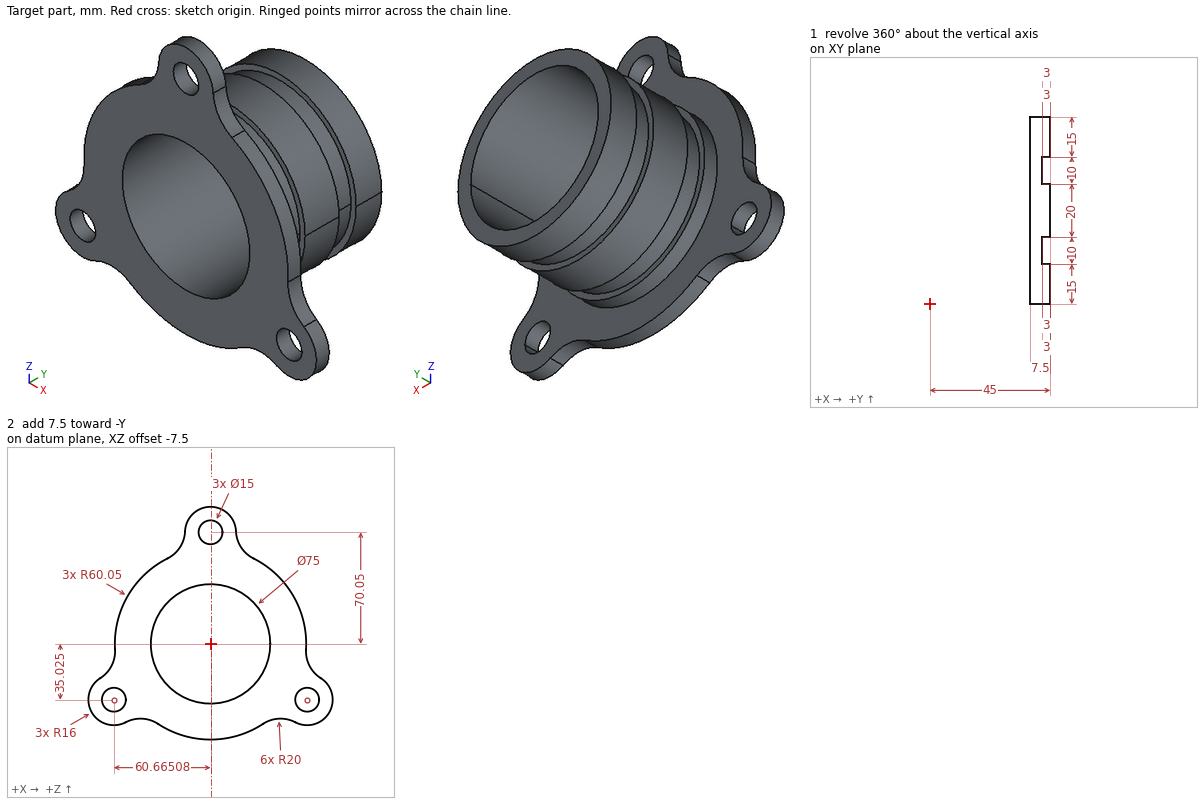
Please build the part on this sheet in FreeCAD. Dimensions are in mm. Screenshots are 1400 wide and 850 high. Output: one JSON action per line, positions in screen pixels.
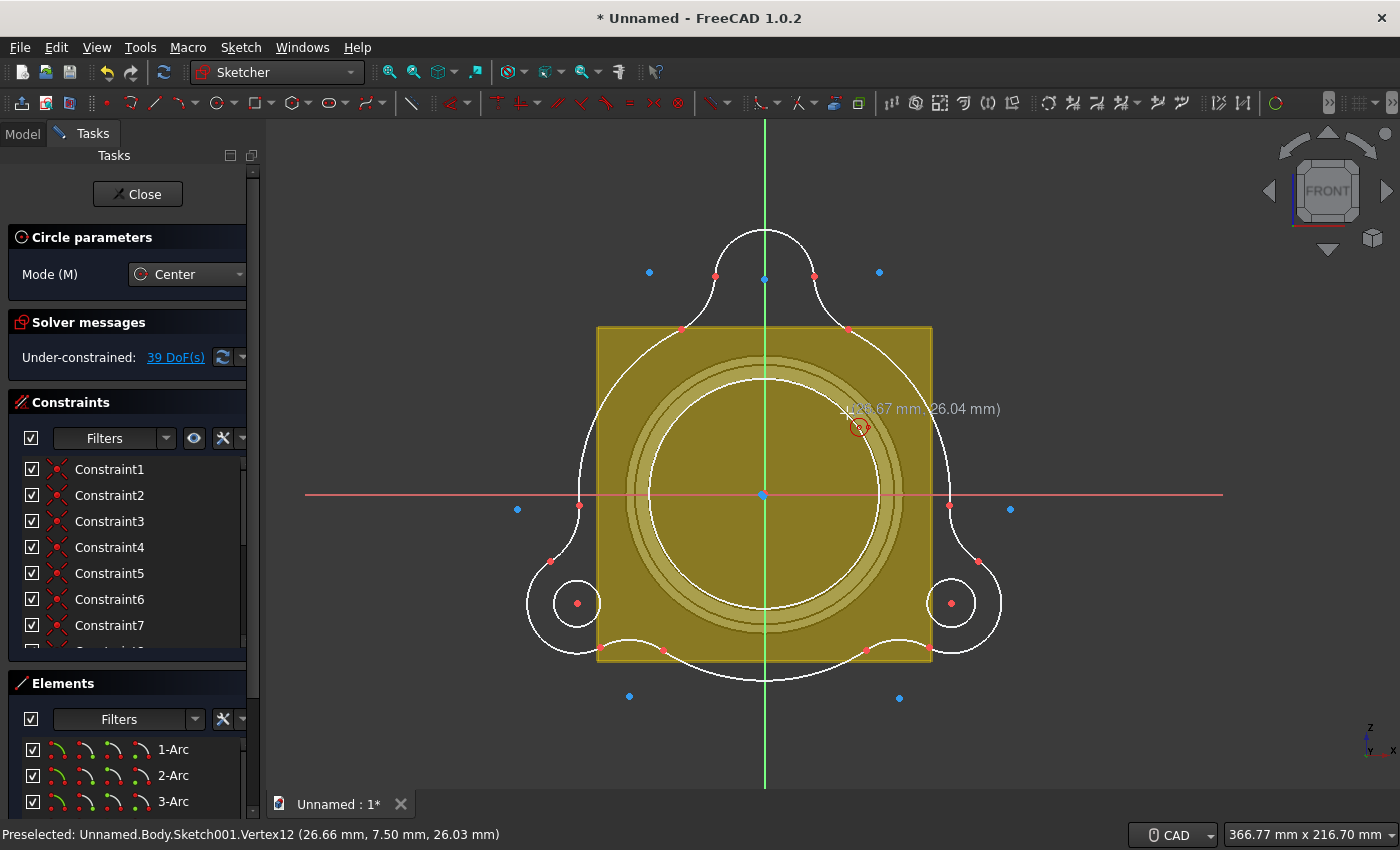
{"action": "left_click", "coordinate": [765, 278]}
{"action": "left_click", "coordinate": [781, 262]}
{"action": "key", "text": "Escape"}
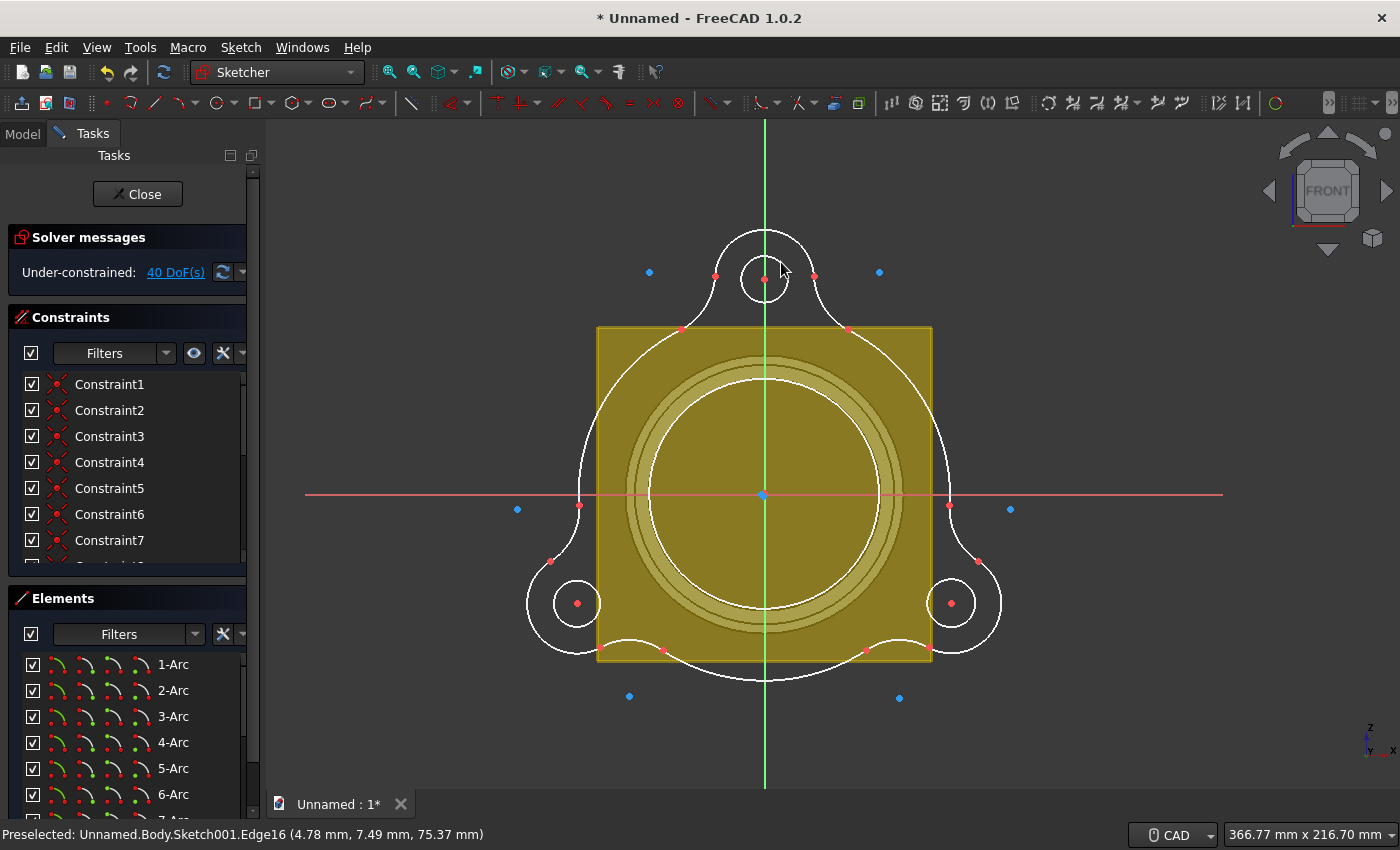
{"action": "left_click", "coordinate": [565, 549]}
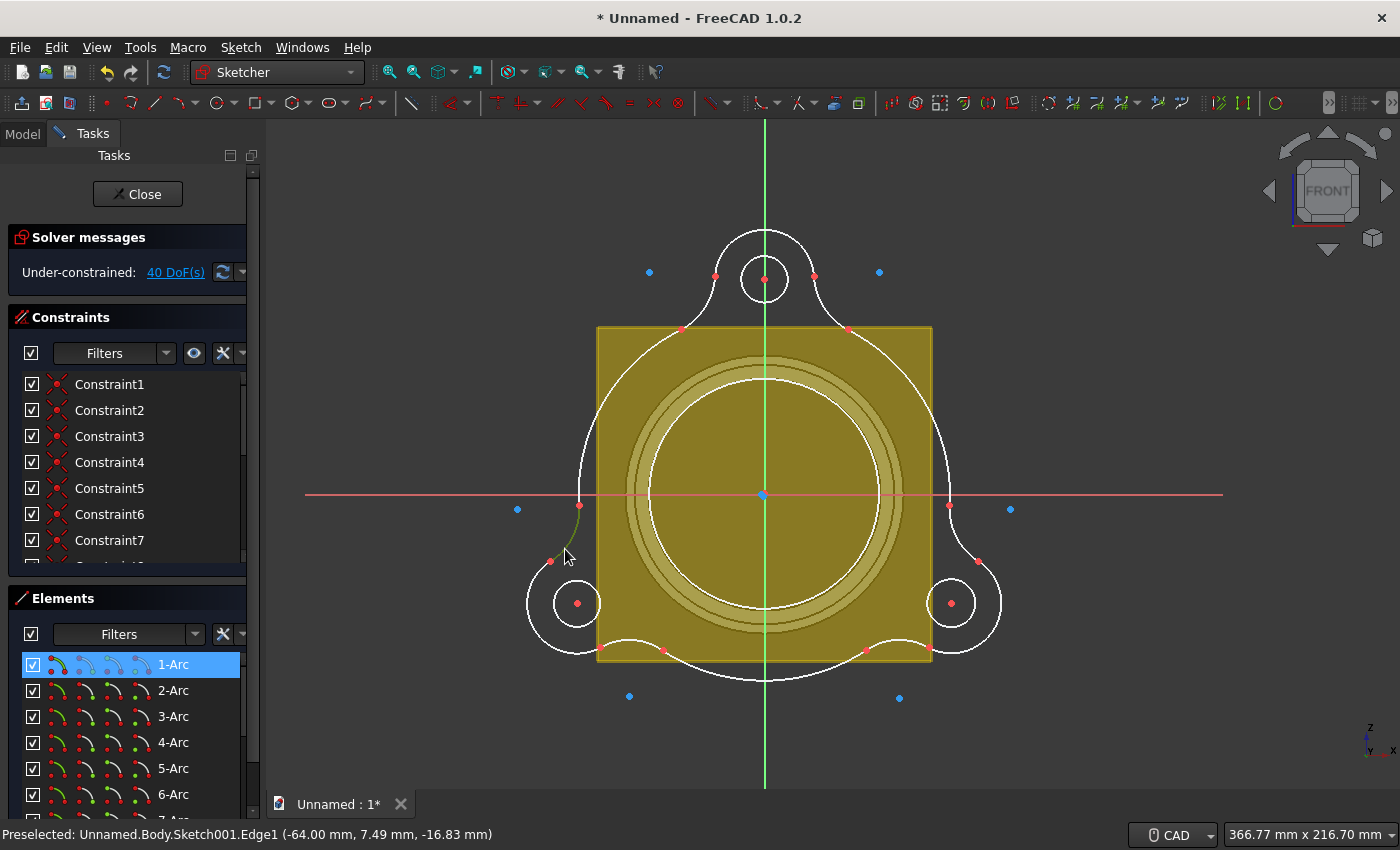
{"action": "left_click", "coordinate": [527, 599]}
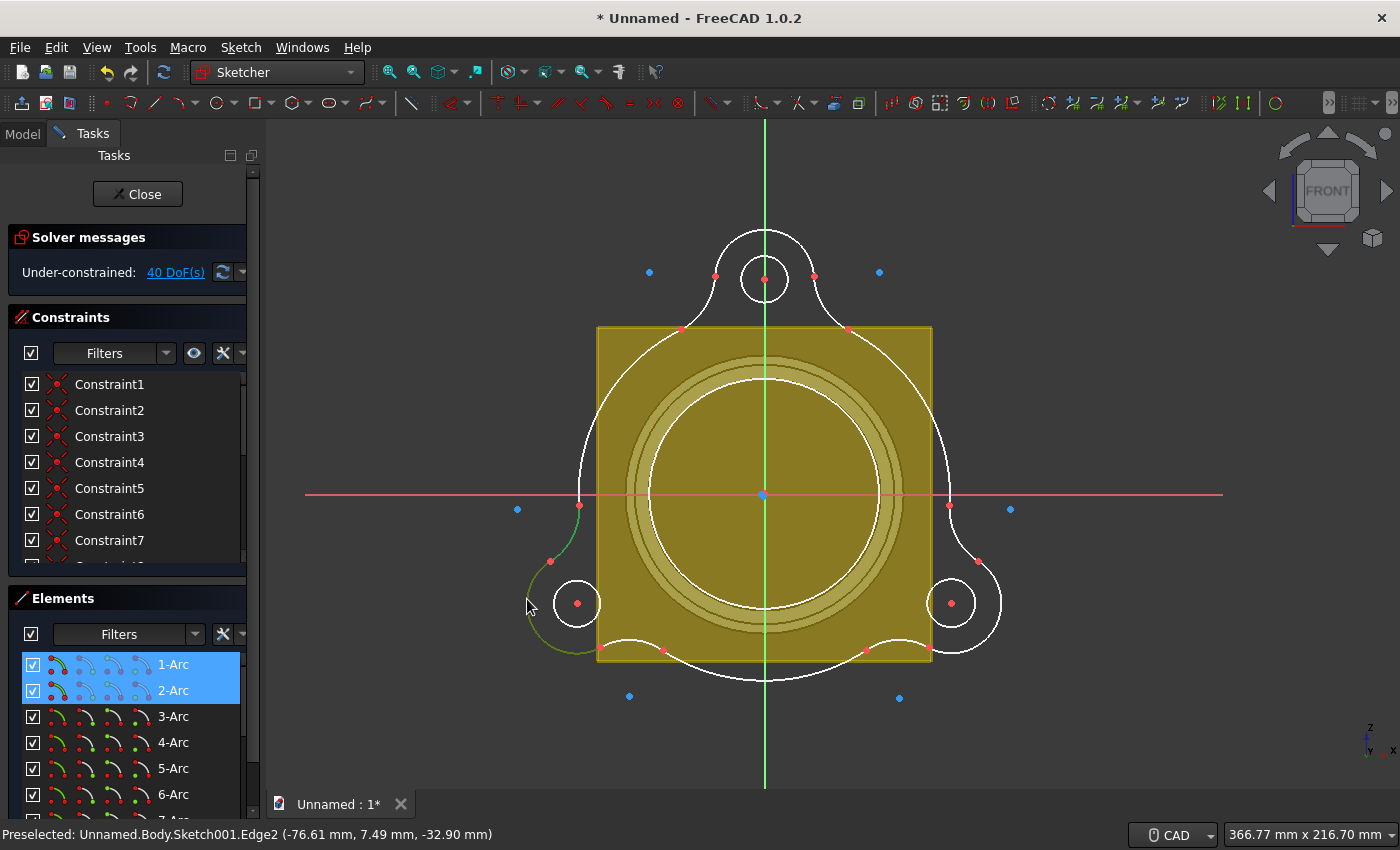
{"action": "left_click", "coordinate": [606, 104]}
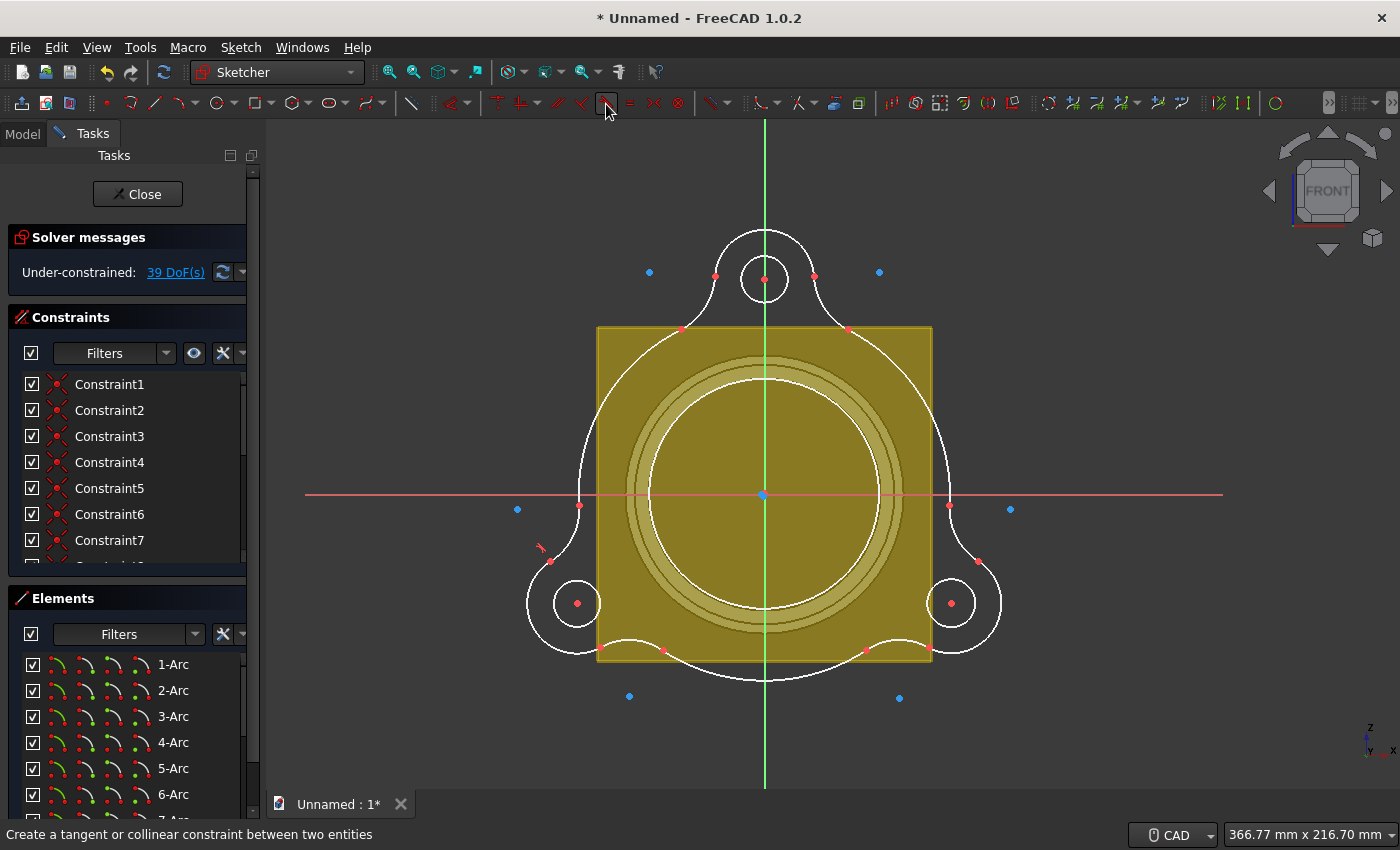
{"action": "left_click", "coordinate": [565, 549]}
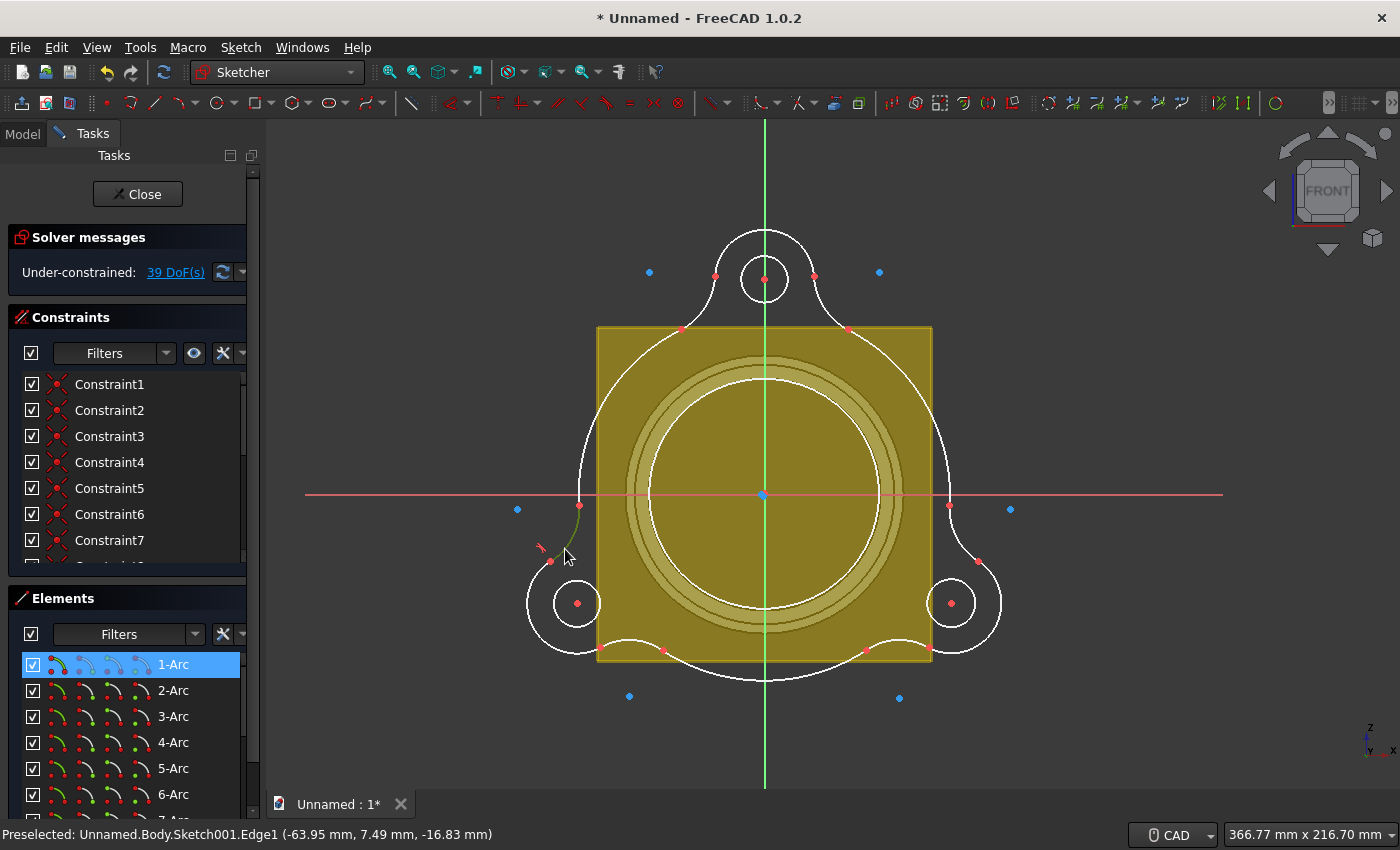
{"action": "left_click", "coordinate": [629, 368]}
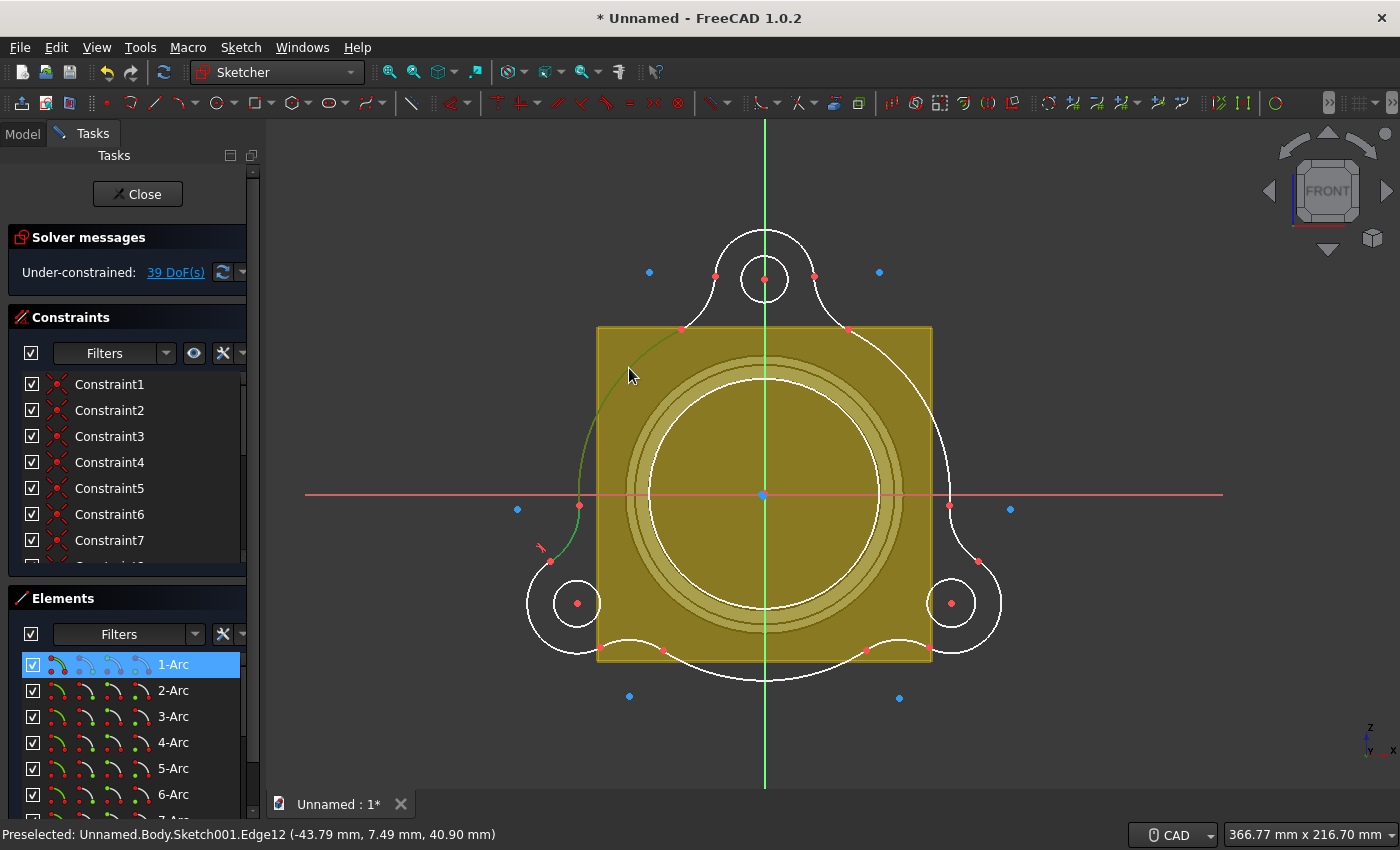
{"action": "key", "text": "t"}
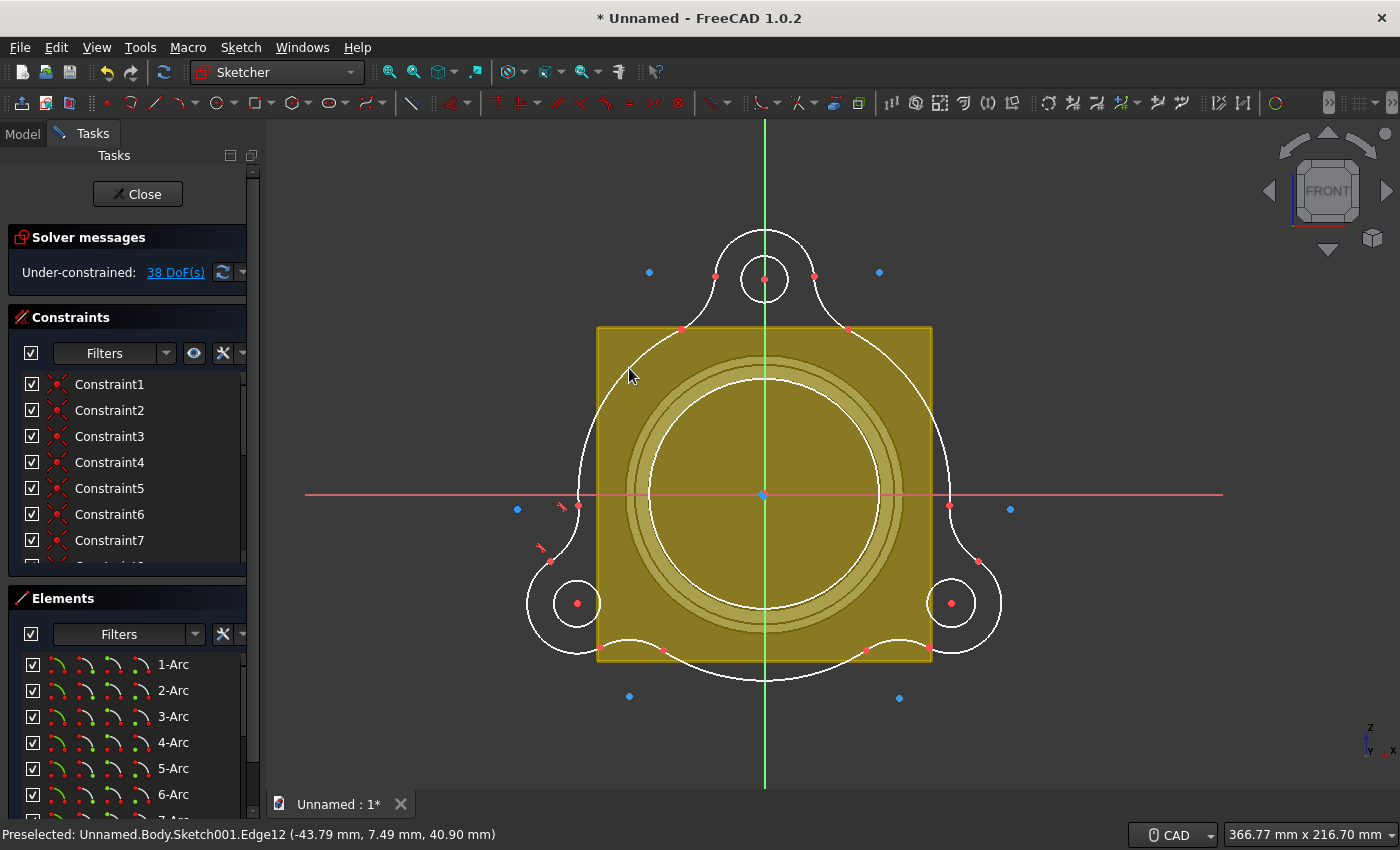
{"action": "left_click", "coordinate": [527, 599]}